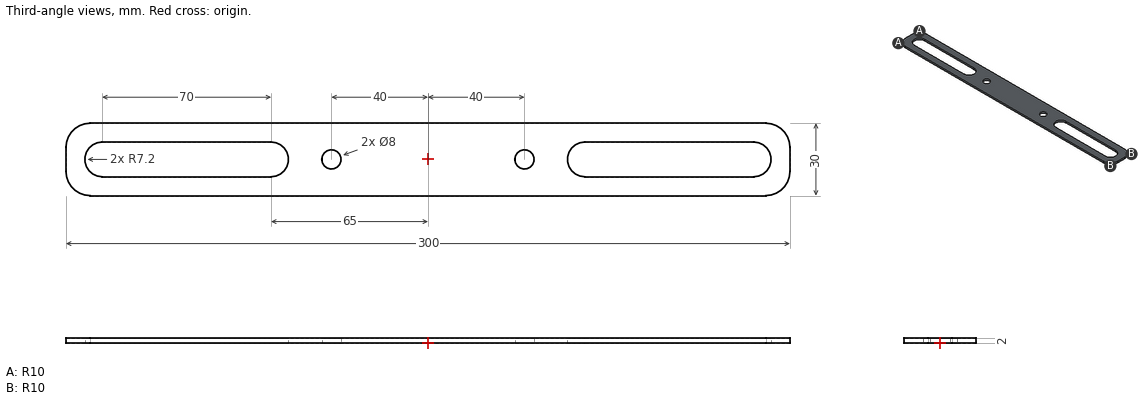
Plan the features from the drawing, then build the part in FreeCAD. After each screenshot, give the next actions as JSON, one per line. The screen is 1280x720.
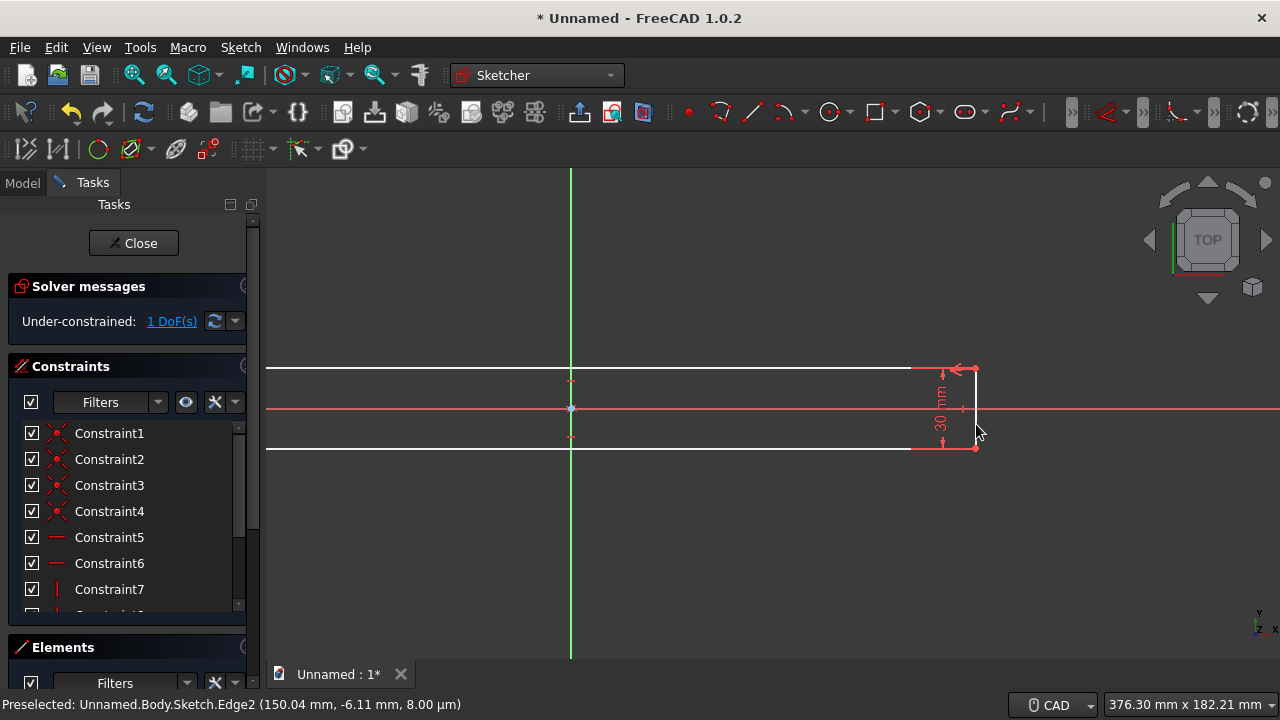
{"action": "left_click", "coordinate": [410, 449]}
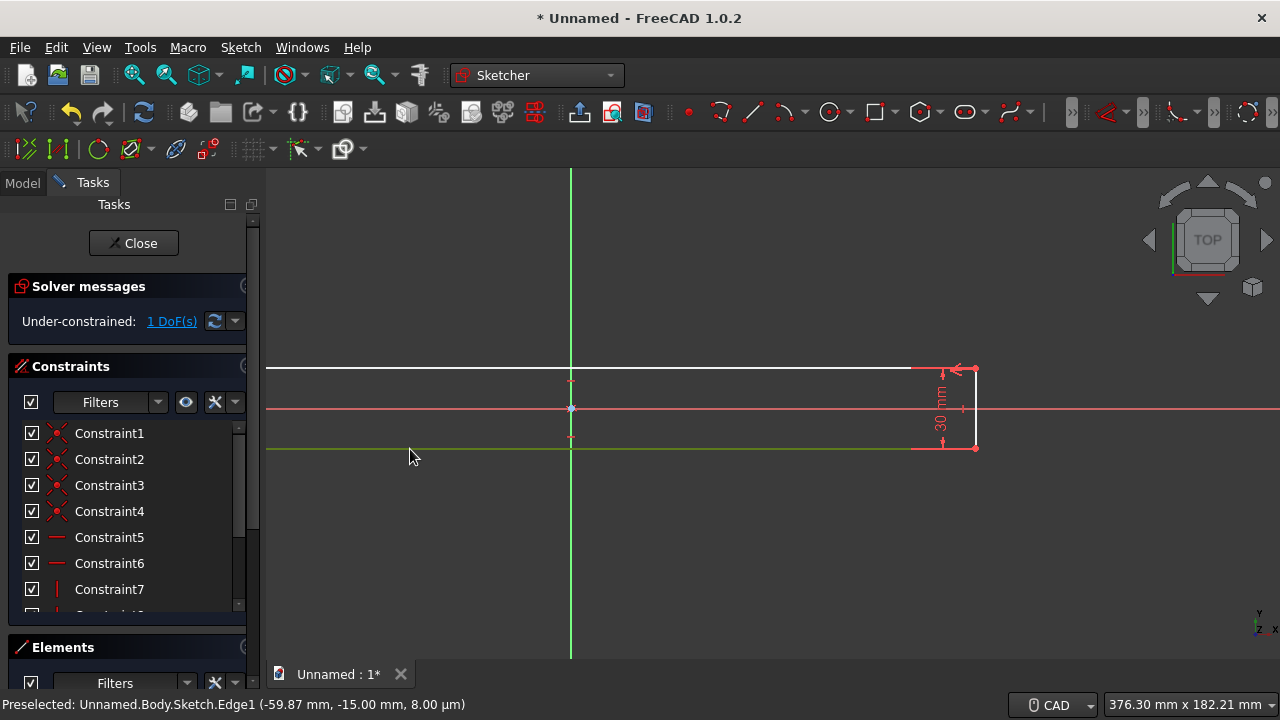
{"action": "key", "text": "l"}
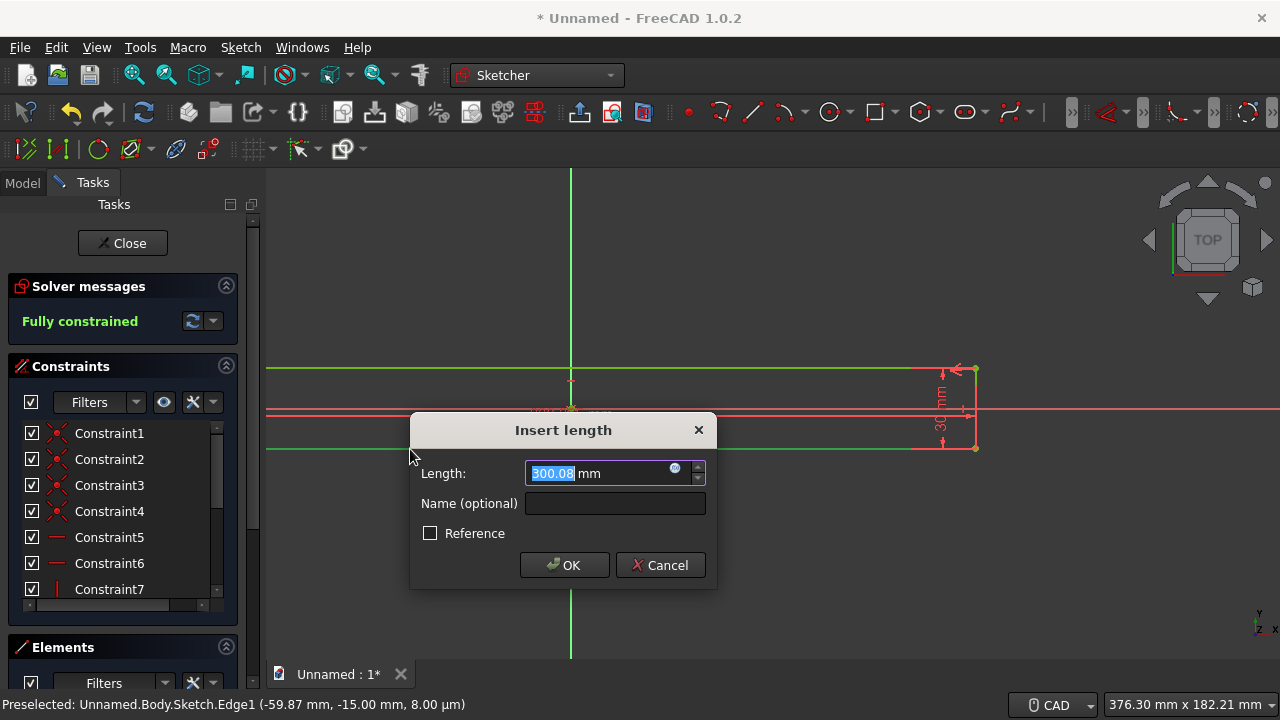
{"action": "type", "text": "300"}
{"action": "key", "text": "Return"}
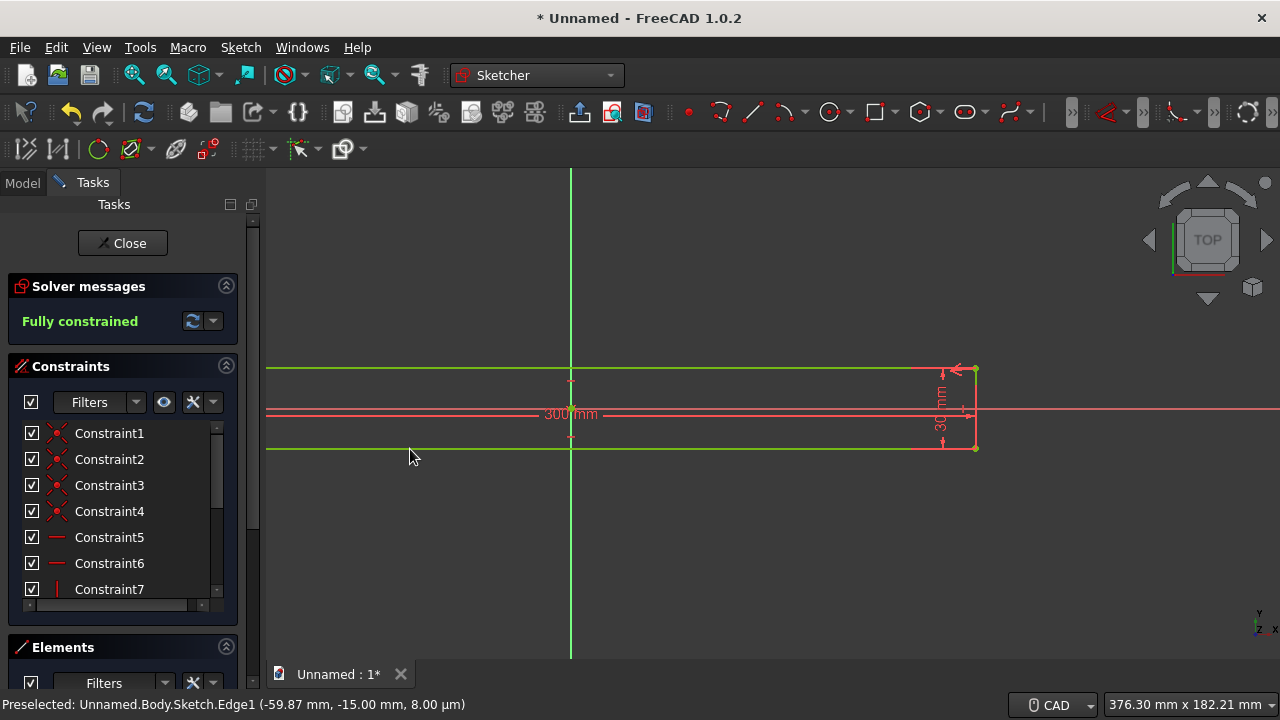
{"action": "left_click", "coordinate": [123, 243]}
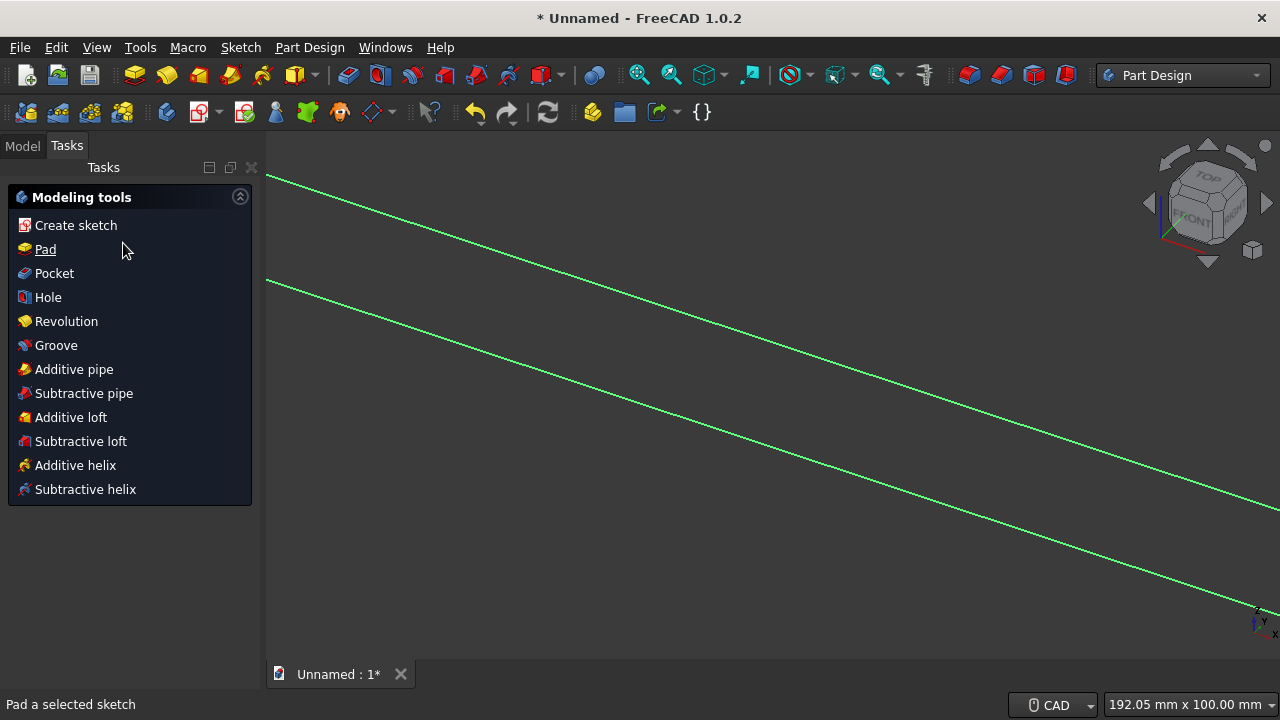
{"action": "left_click", "coordinate": [136, 76]}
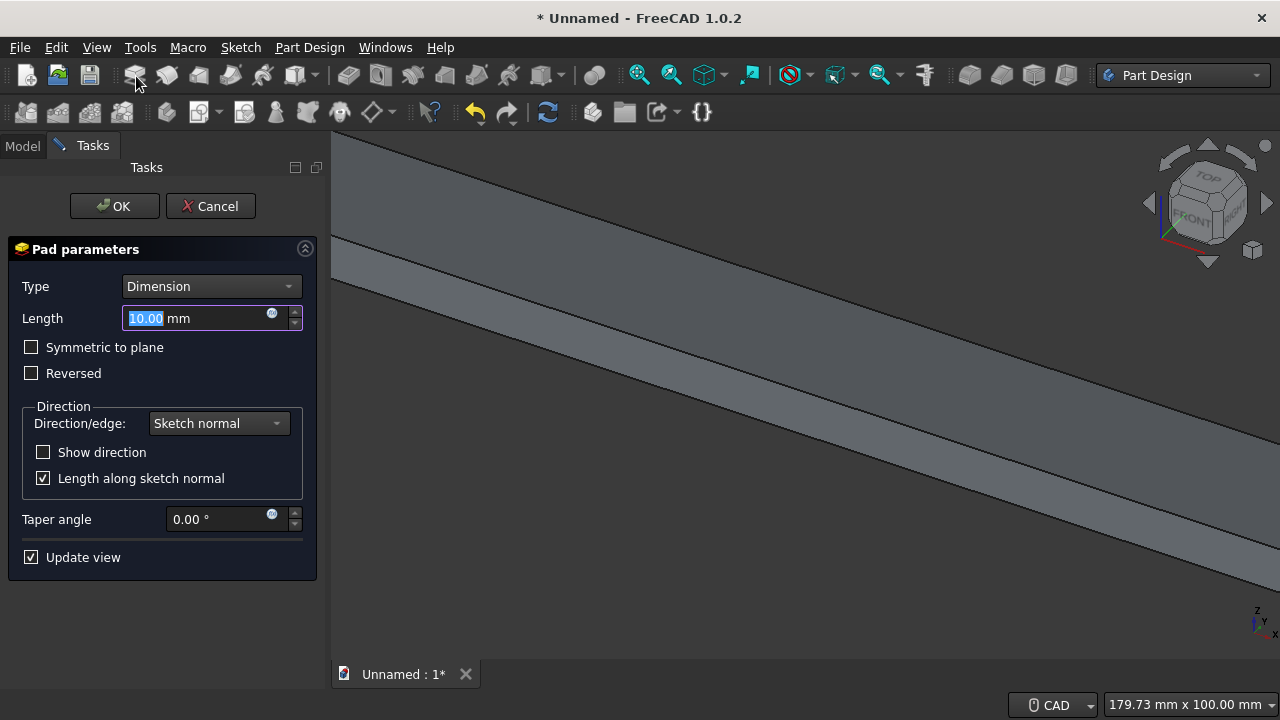
{"action": "type", "text": "2"}
{"action": "key", "text": "Tab"}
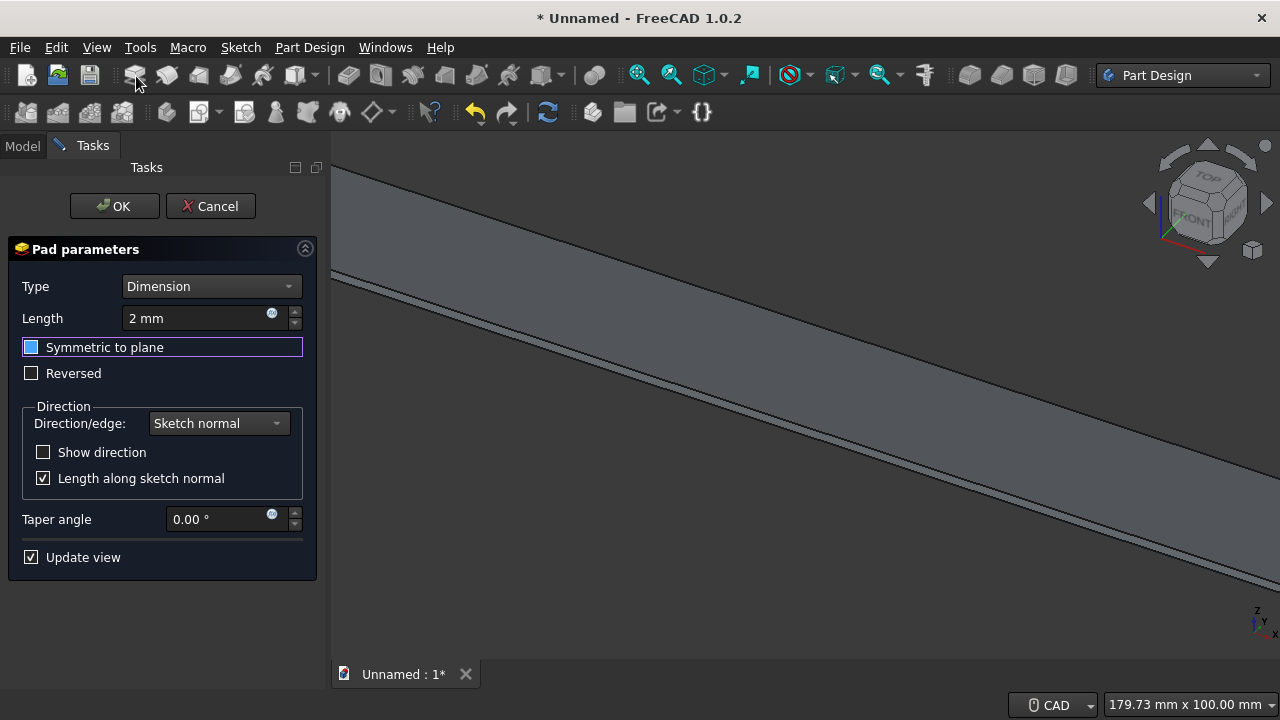
{"action": "left_click", "coordinate": [115, 206]}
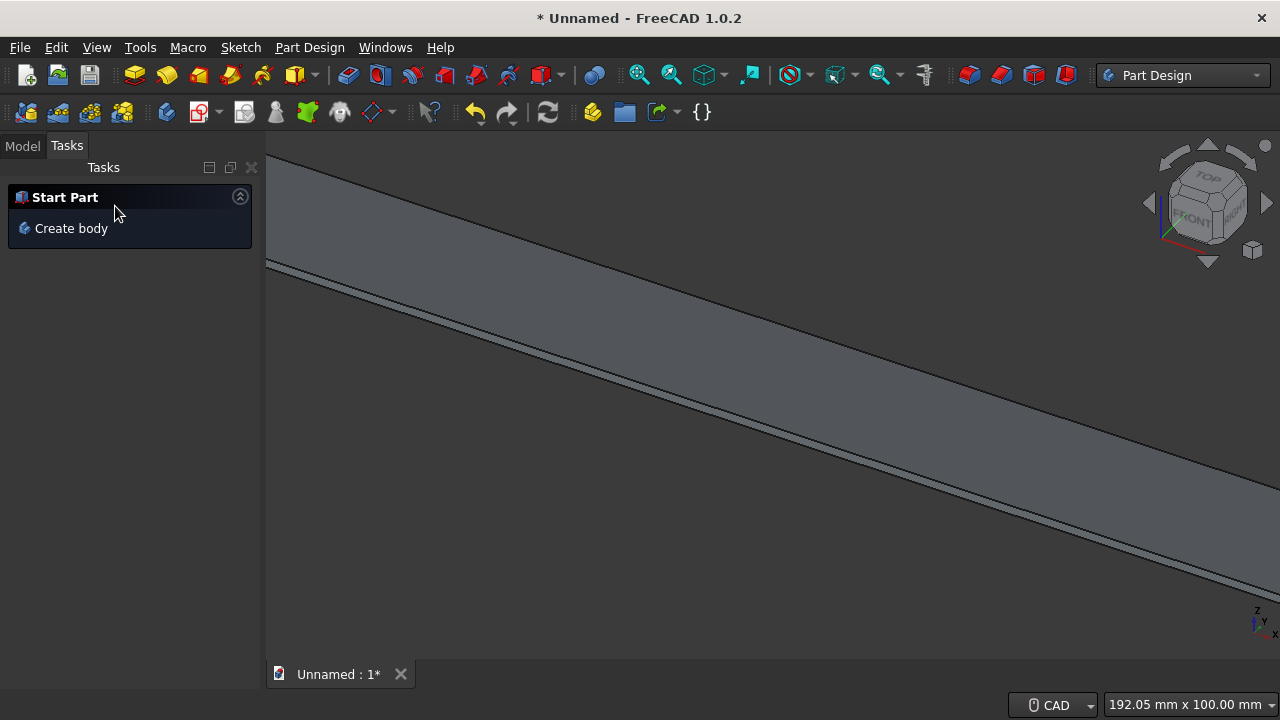
{"action": "key", "text": "v f"}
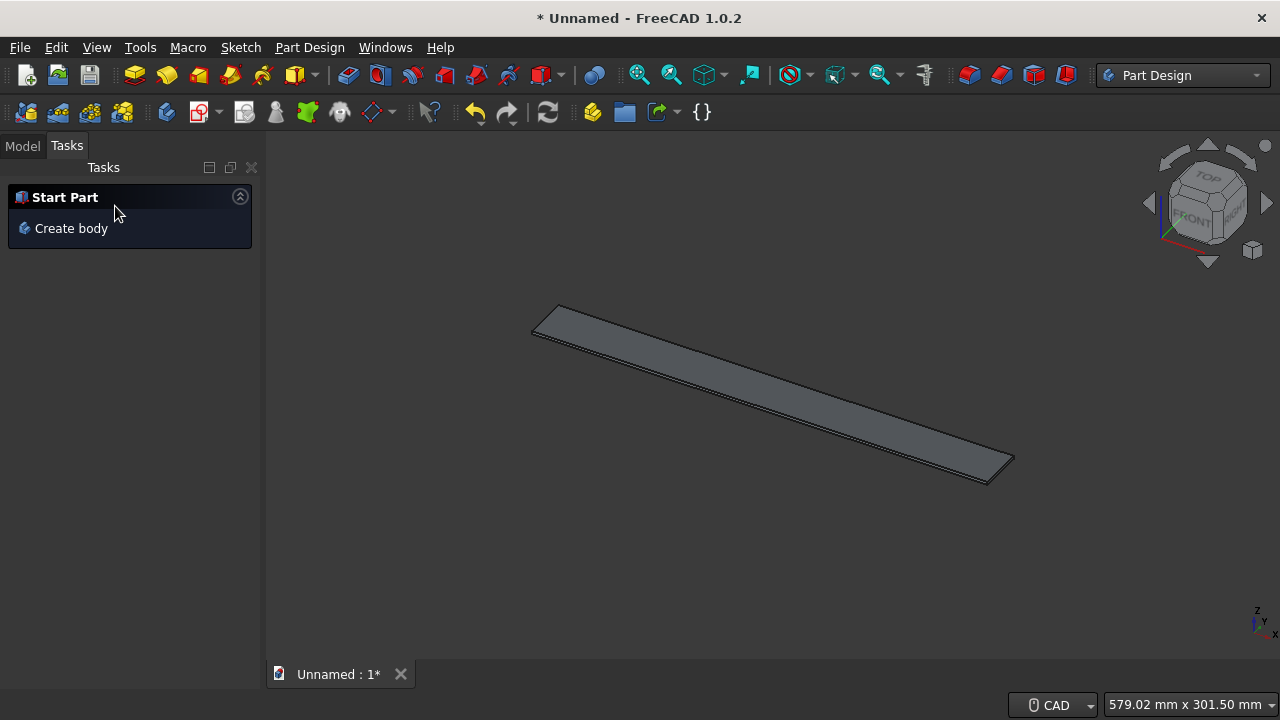
{"action": "left_click", "coordinate": [968, 457]}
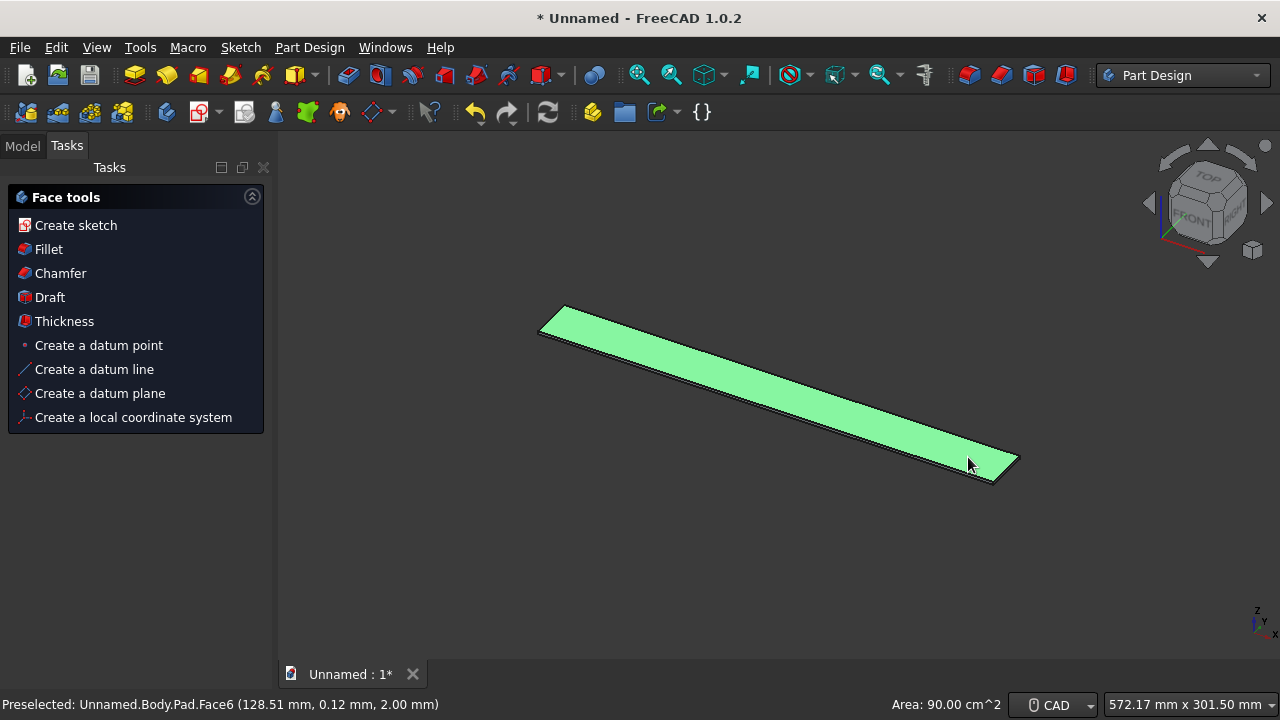
{"action": "left_click", "coordinate": [200, 112]}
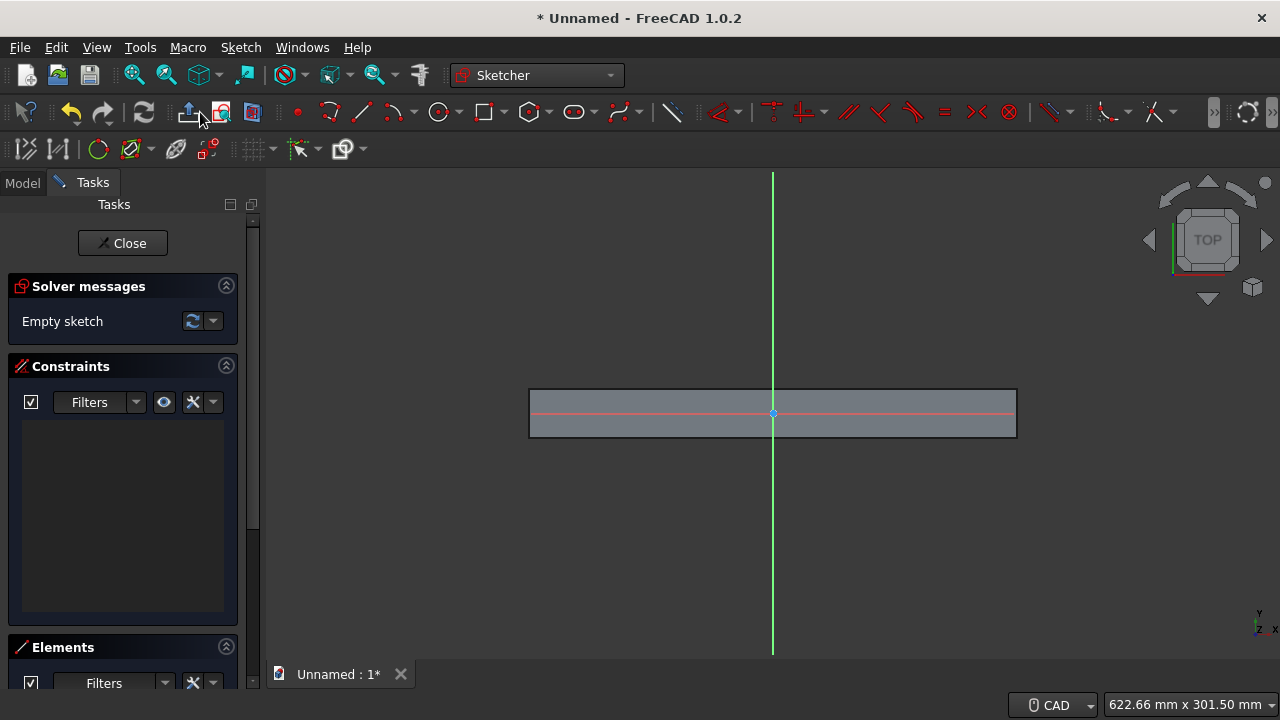
{"action": "scroll", "coordinate": [630, 414], "scroll_direction": "up", "scroll_amount": 5}